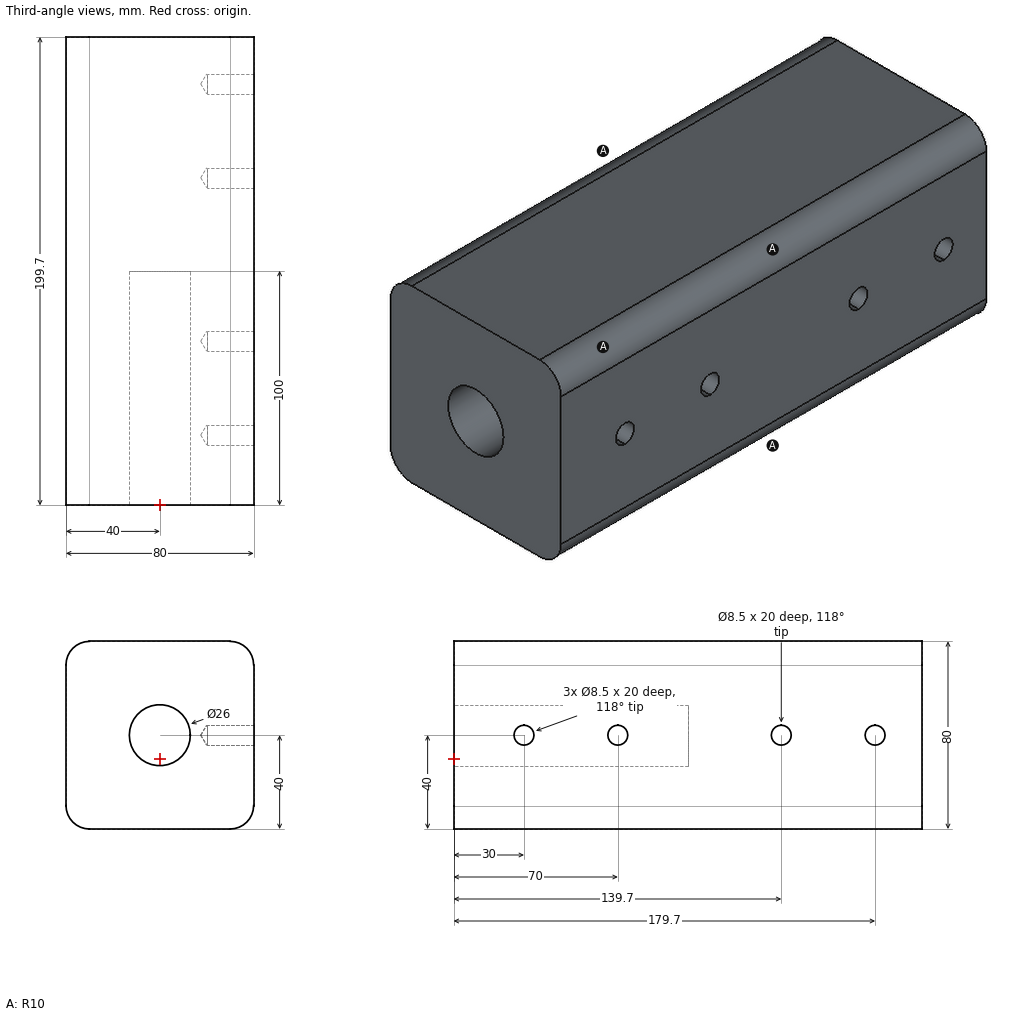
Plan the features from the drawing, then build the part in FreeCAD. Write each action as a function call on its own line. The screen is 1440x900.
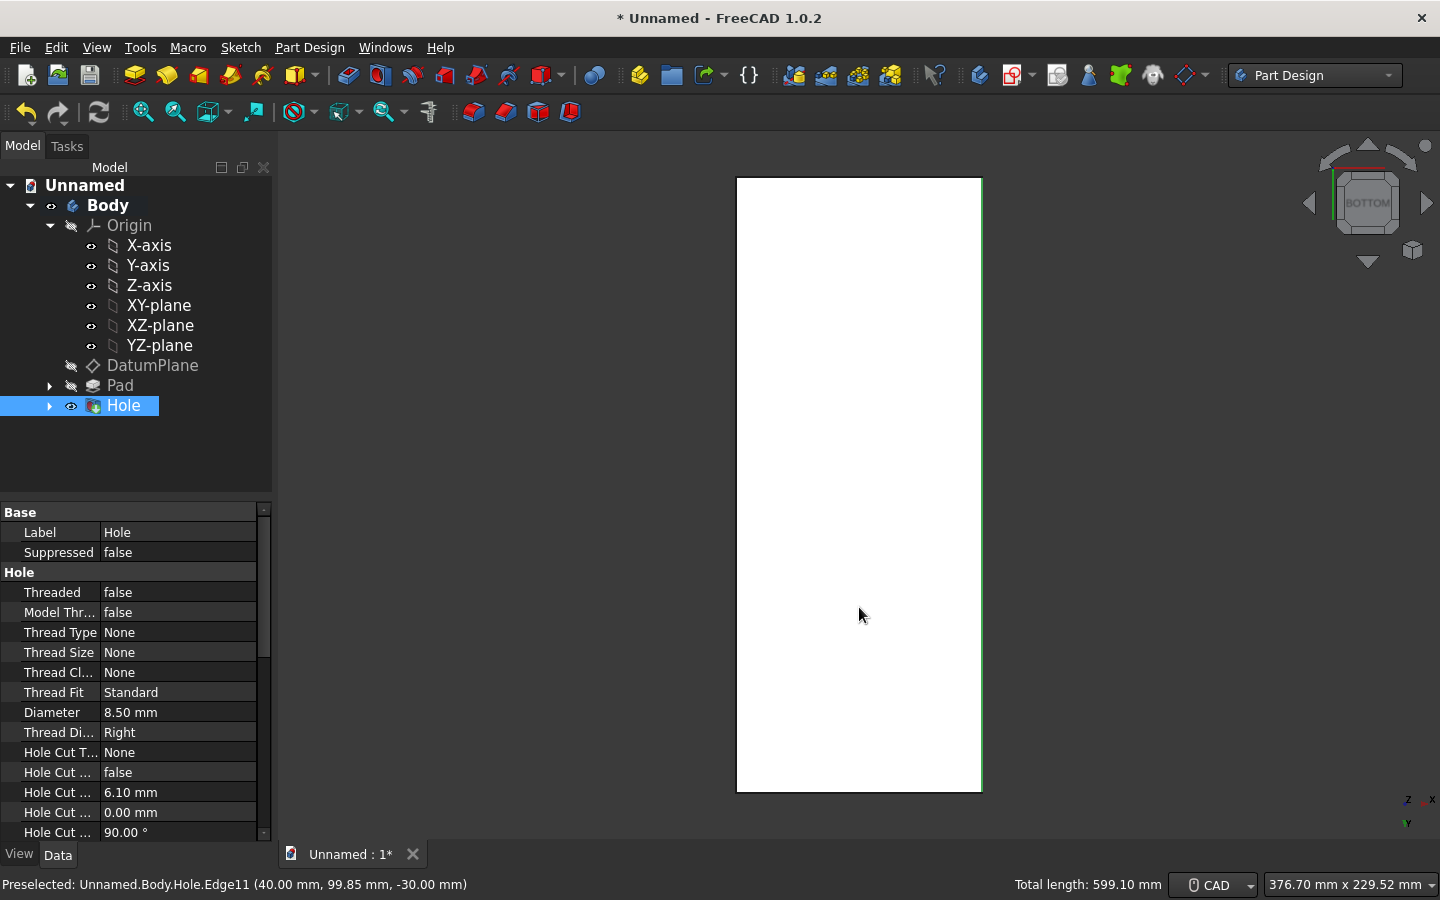
click(736, 484, ctrl)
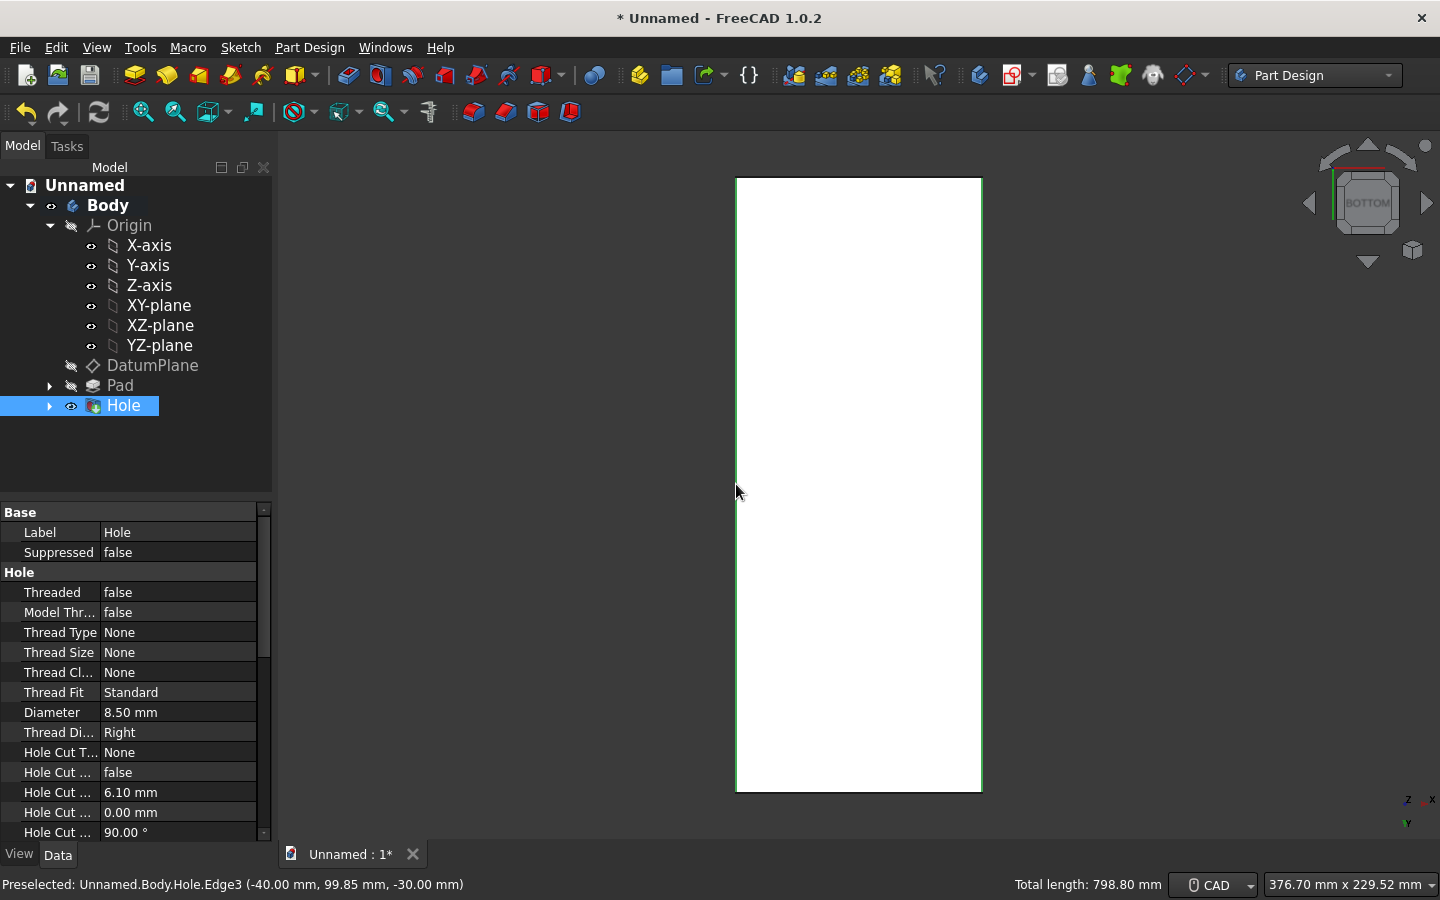
click(474, 112)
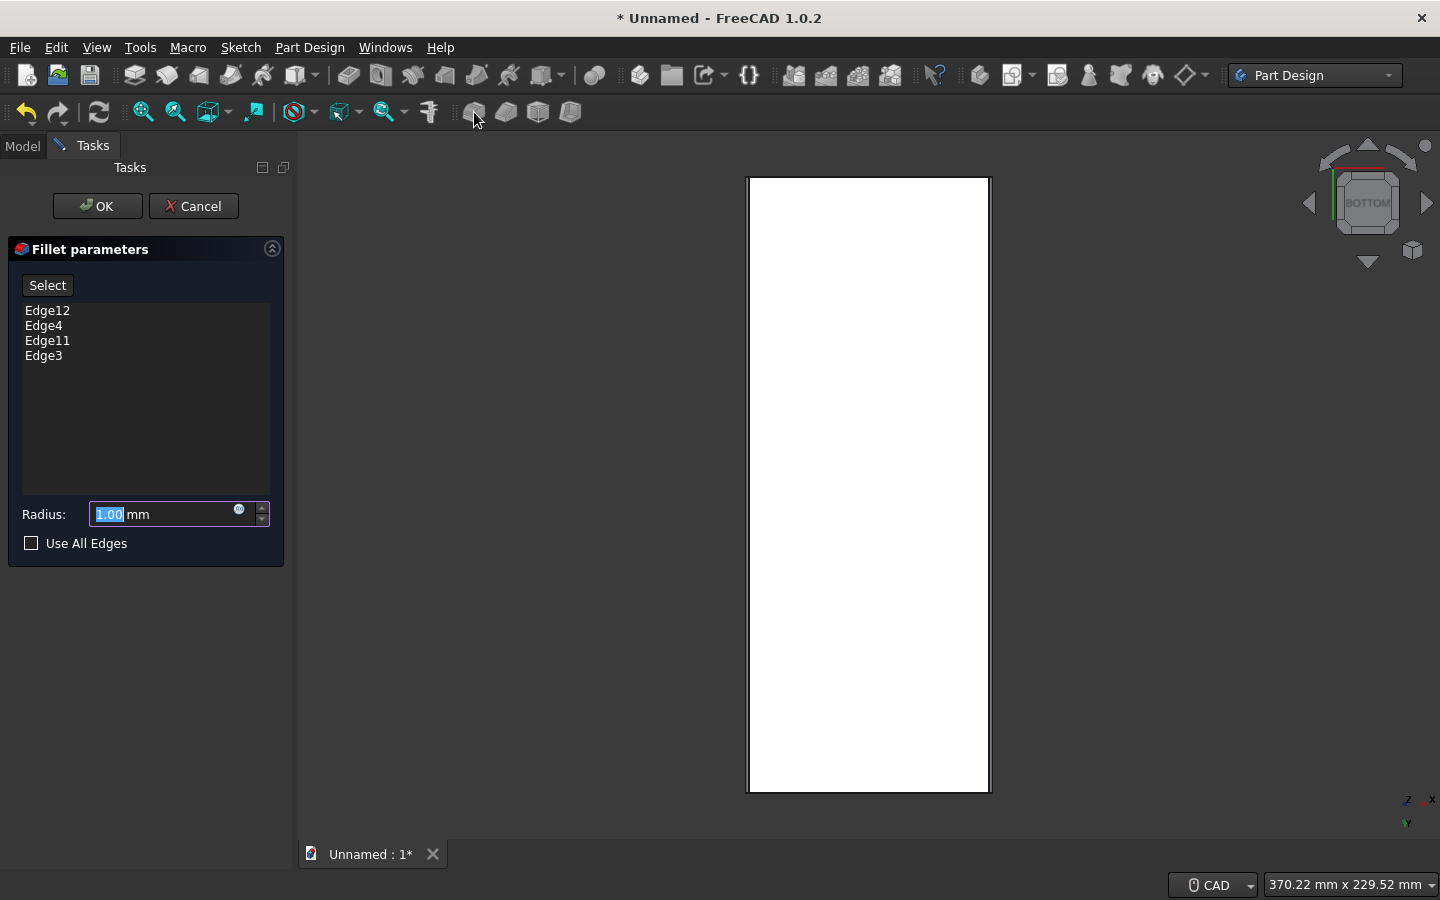
text(10)
key(Tab)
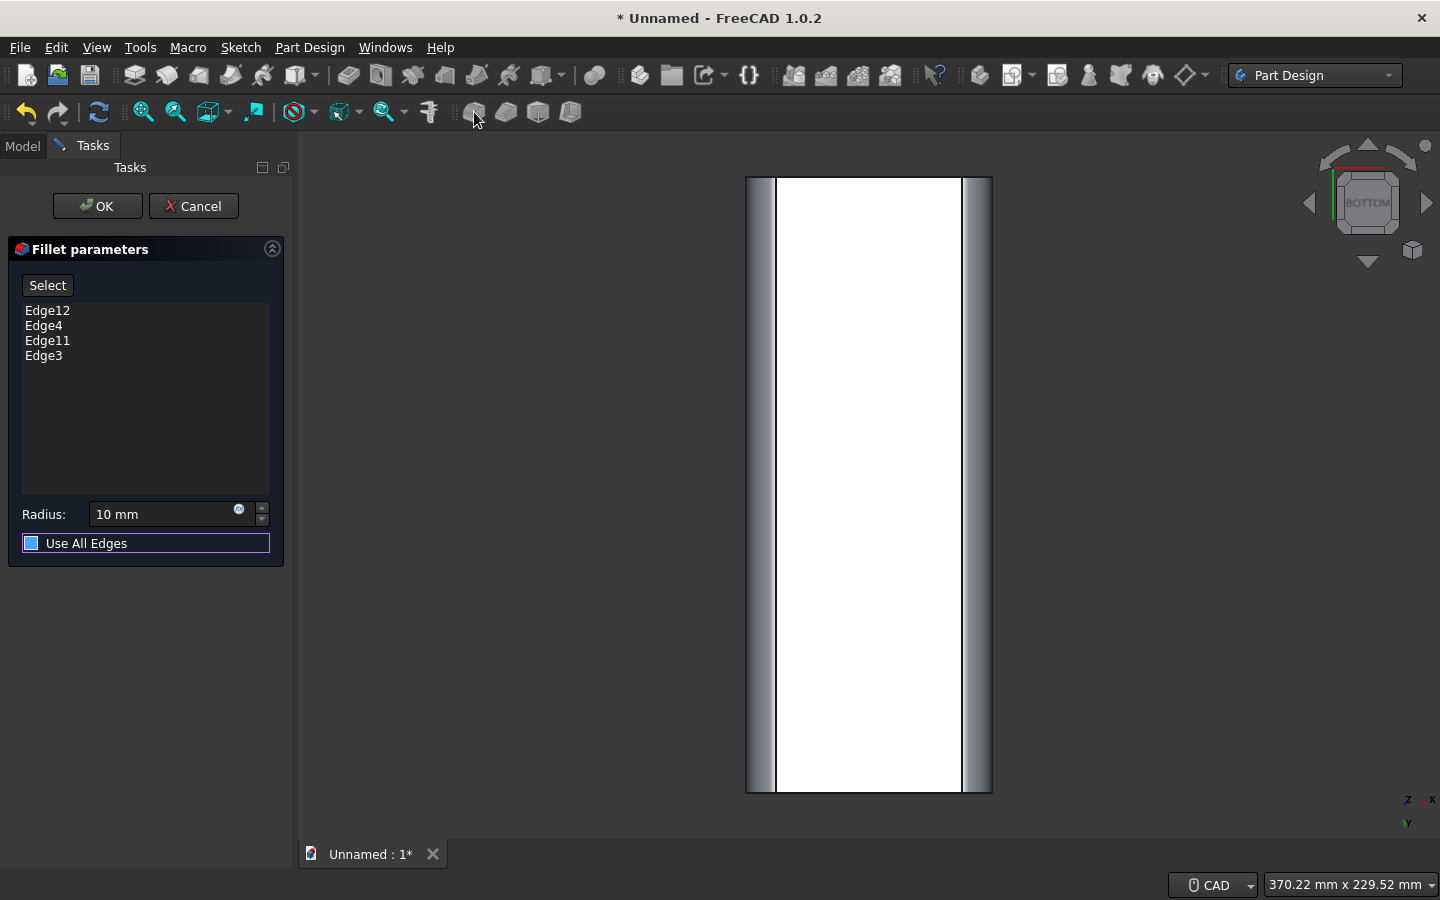
click(98, 206)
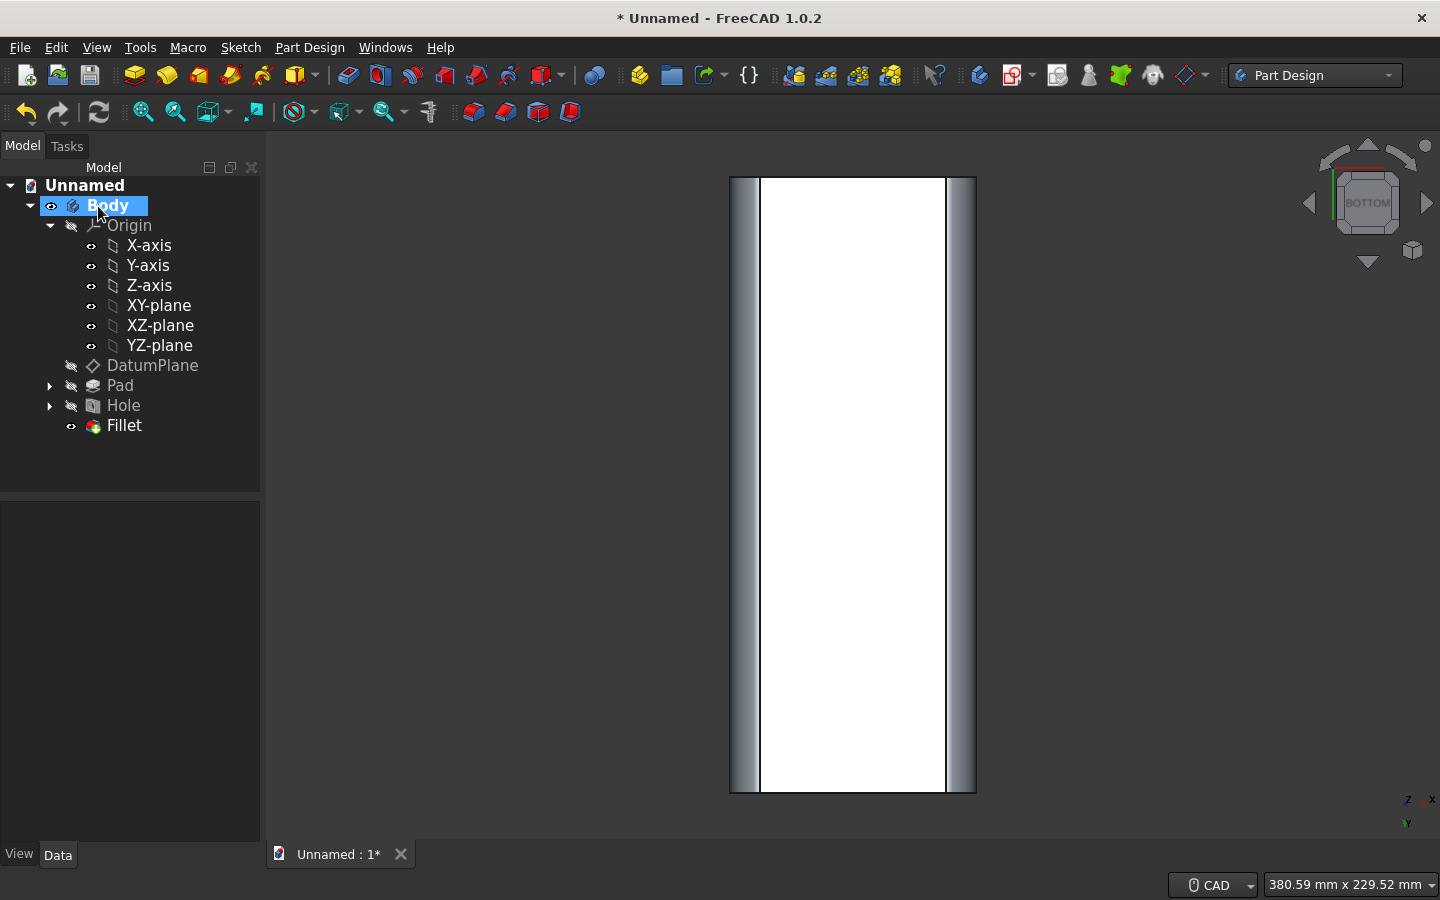
key(0)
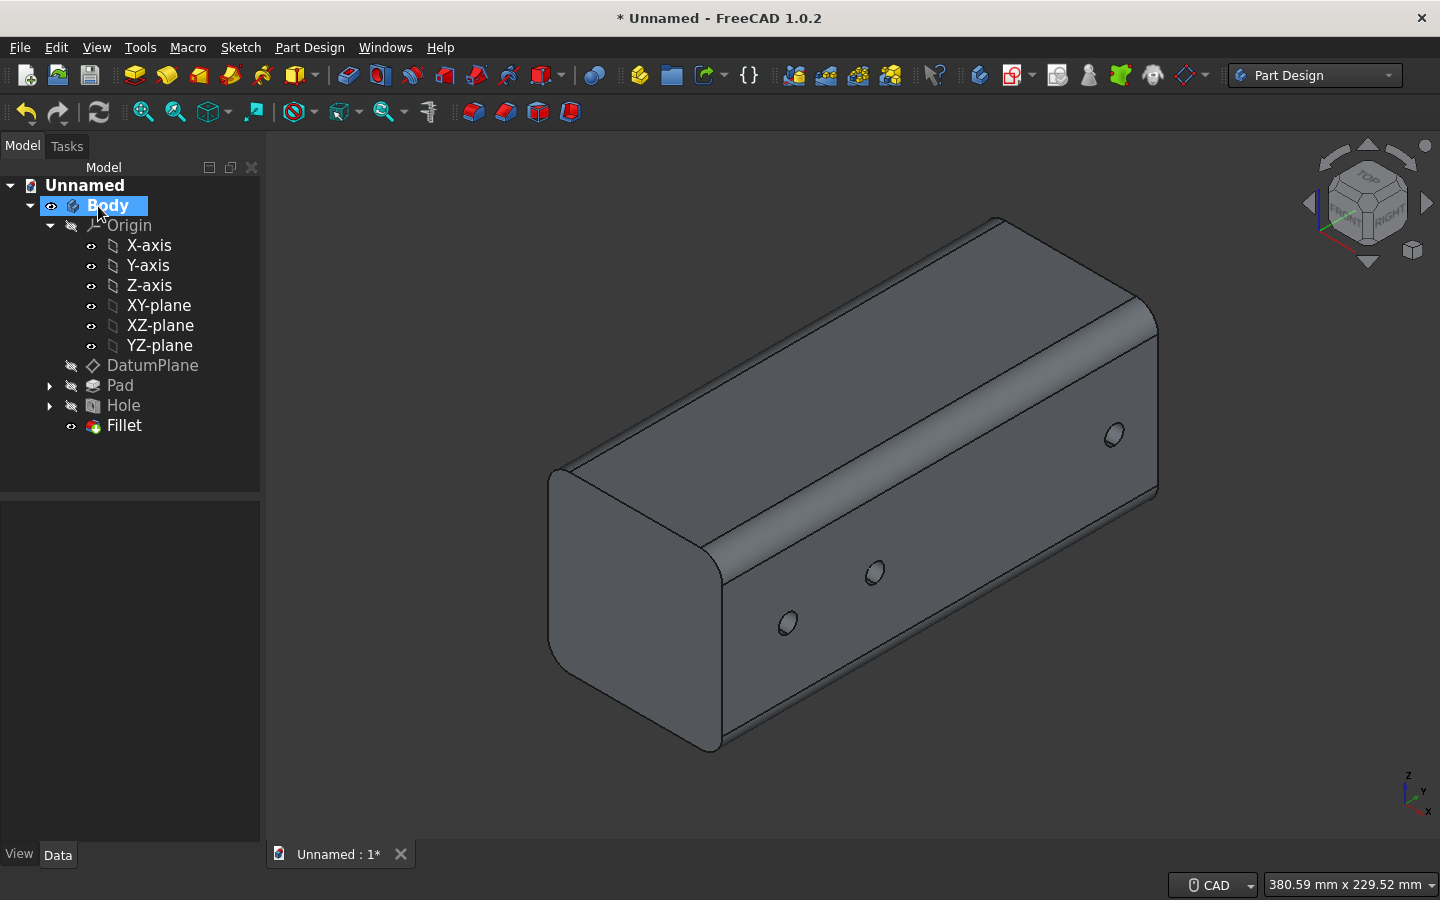
click(635, 610)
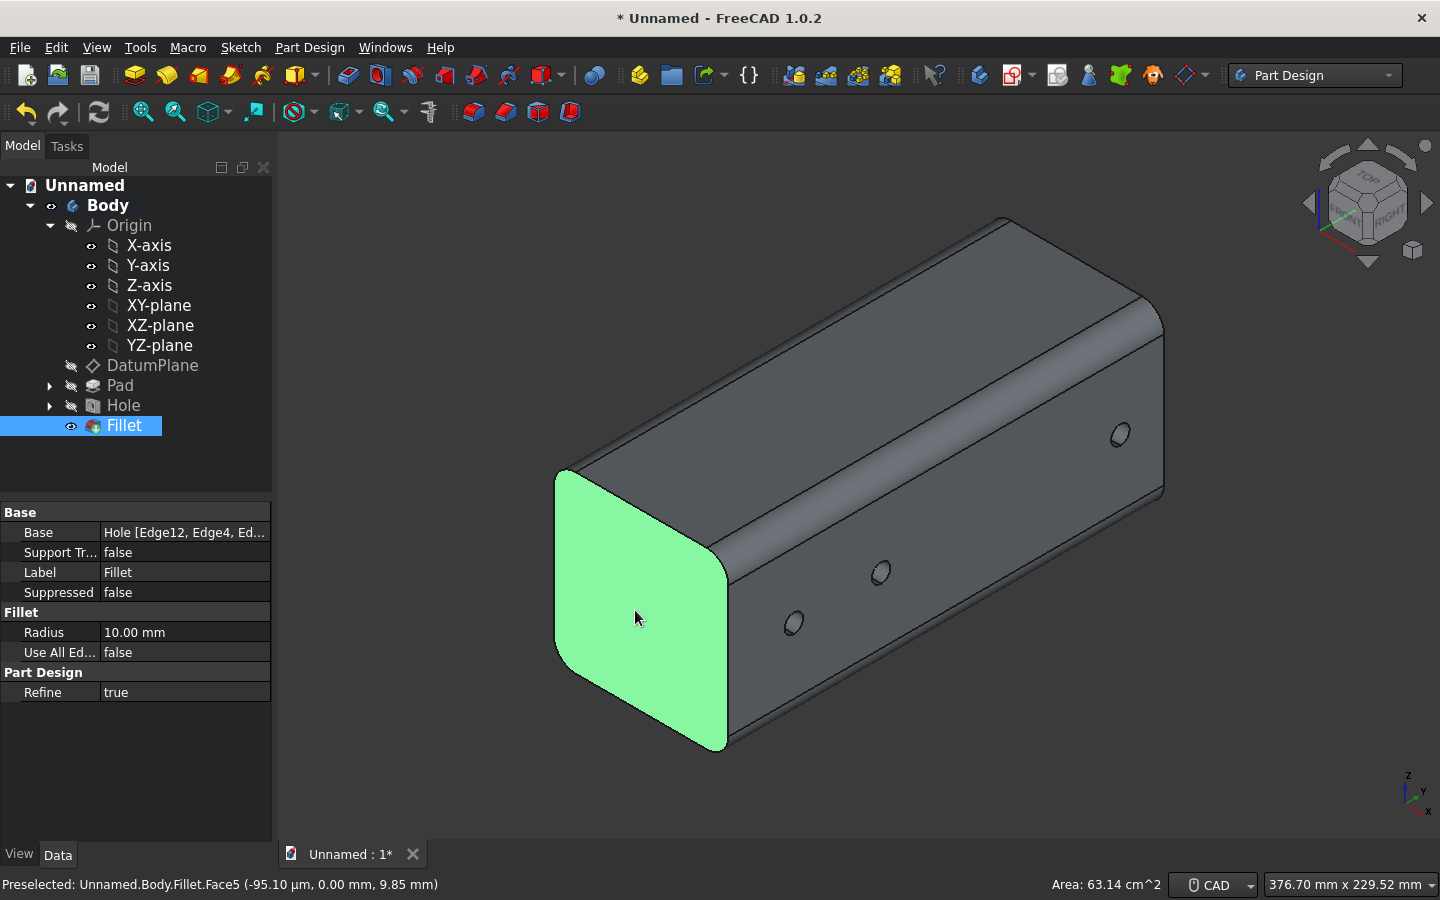
click(1012, 76)